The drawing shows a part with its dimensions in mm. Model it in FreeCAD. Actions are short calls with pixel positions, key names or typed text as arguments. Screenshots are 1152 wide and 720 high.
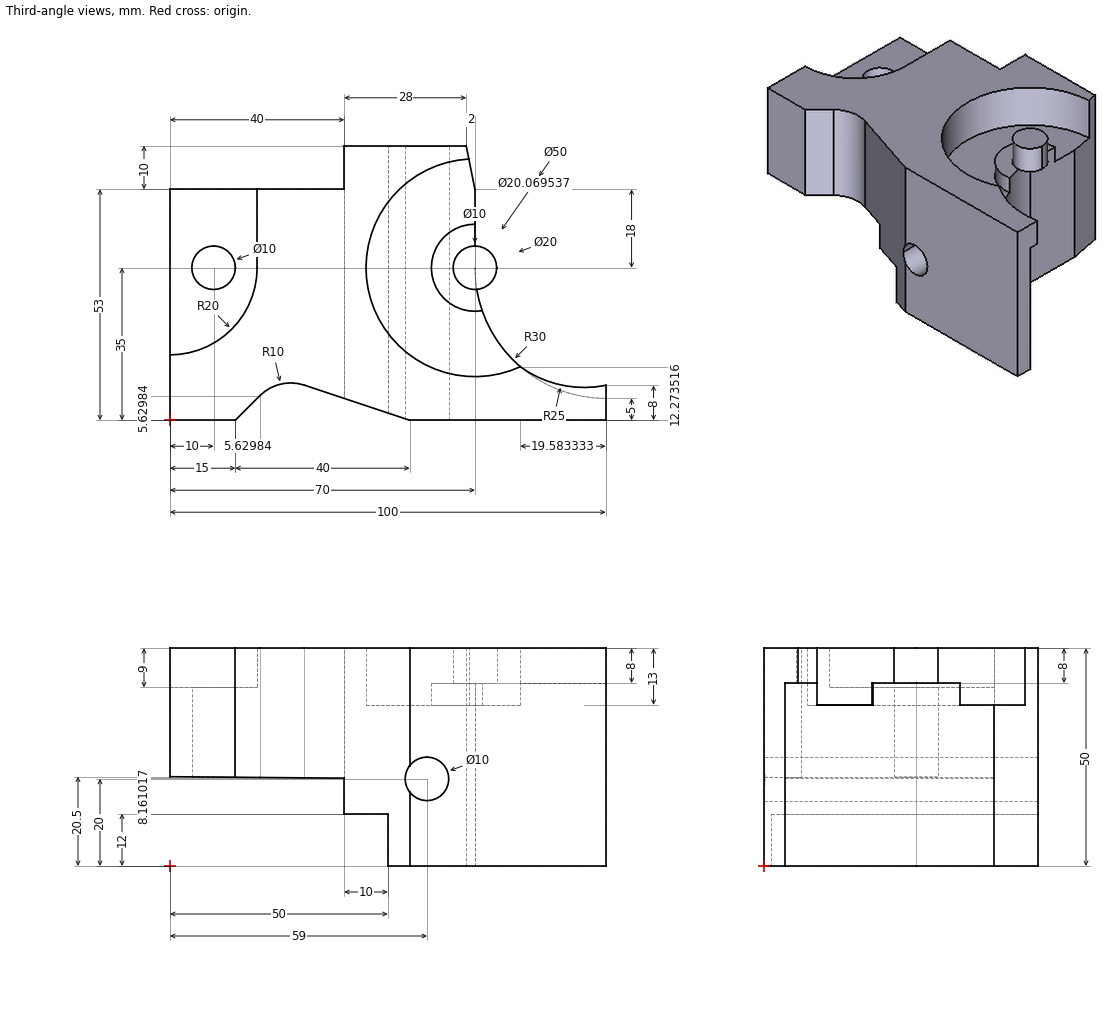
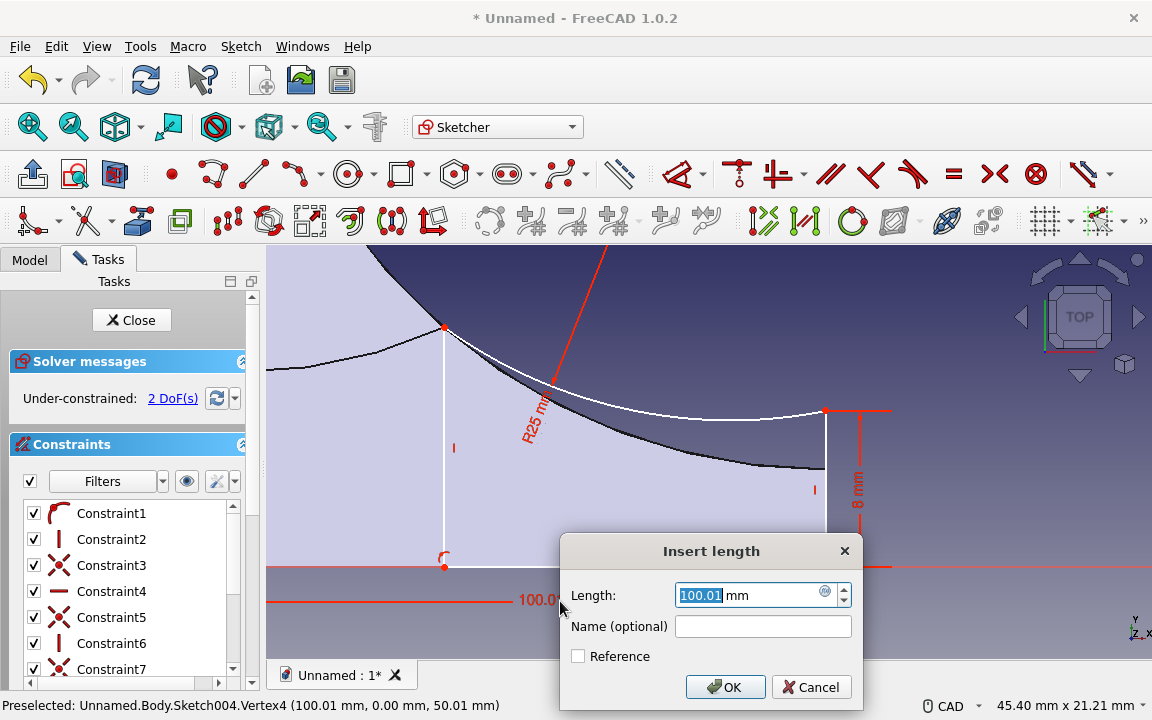
text(100)
key(Return)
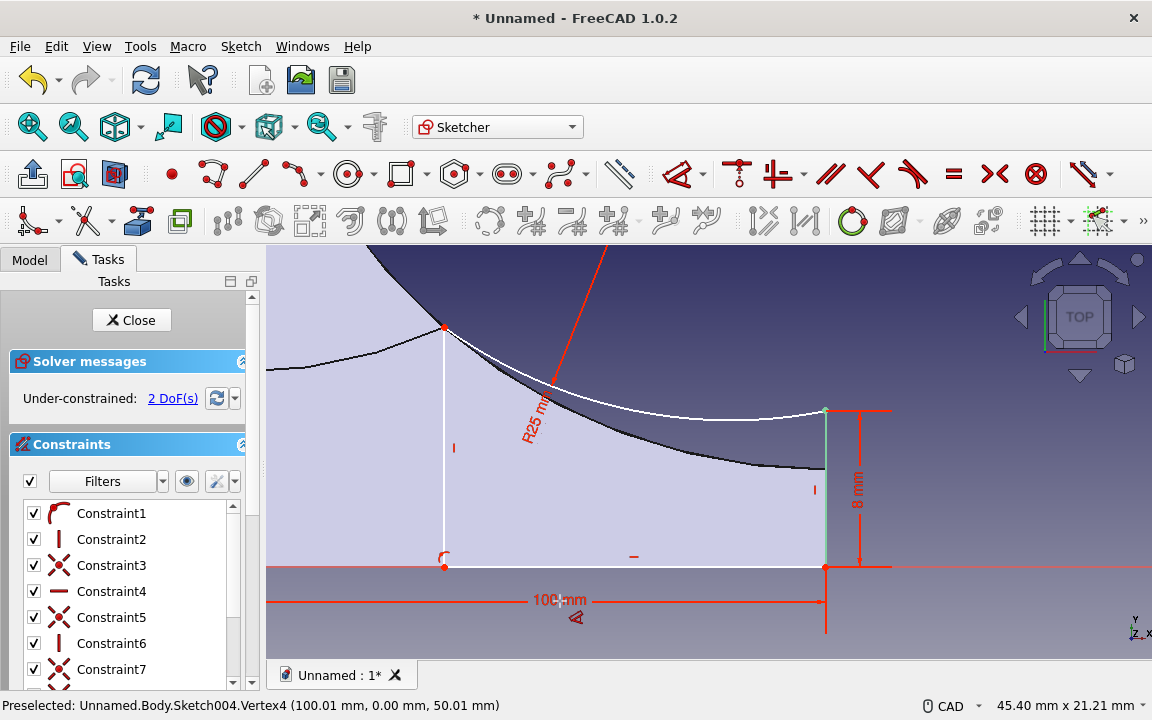
click(444, 399)
click(410, 447)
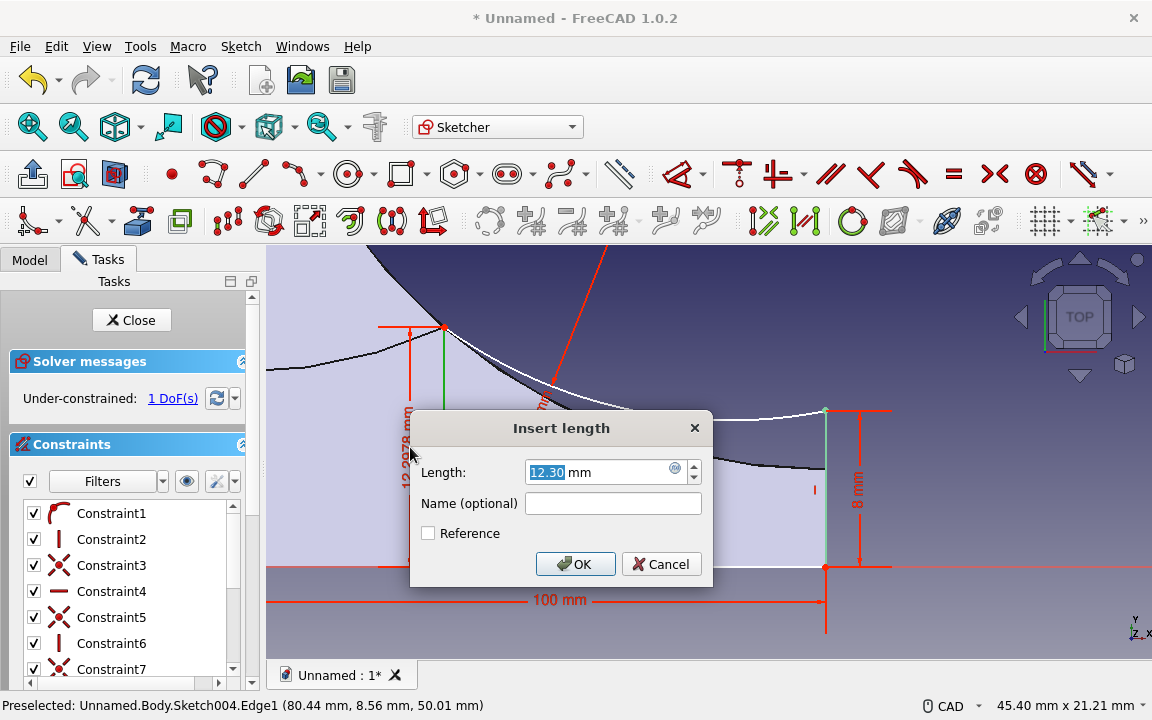
text(12.273516)
key(Return)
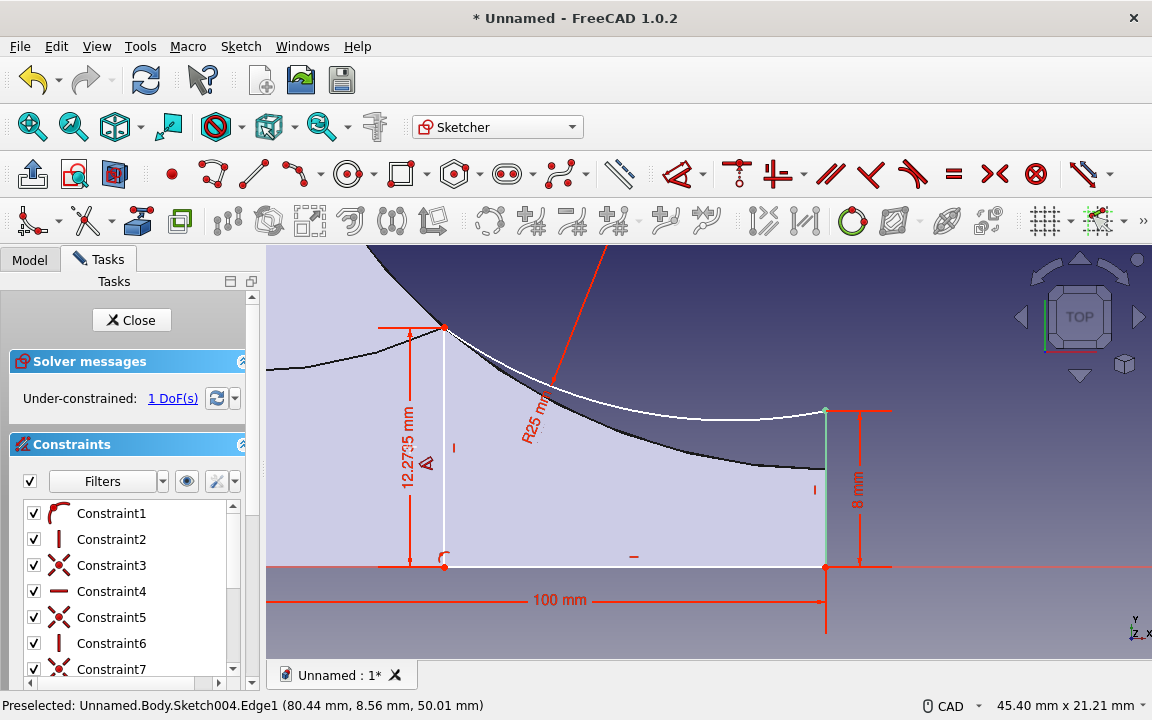
click(559, 567)
click(635, 601)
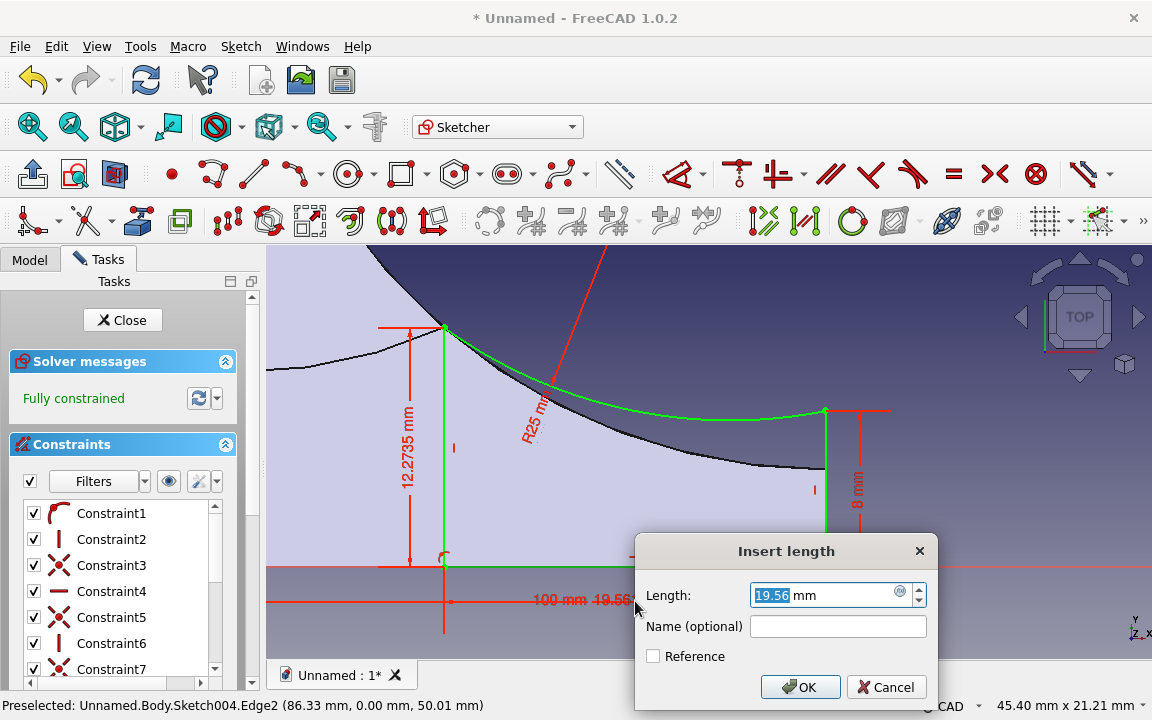
text(19.583333)
key(Return)
key(Escape)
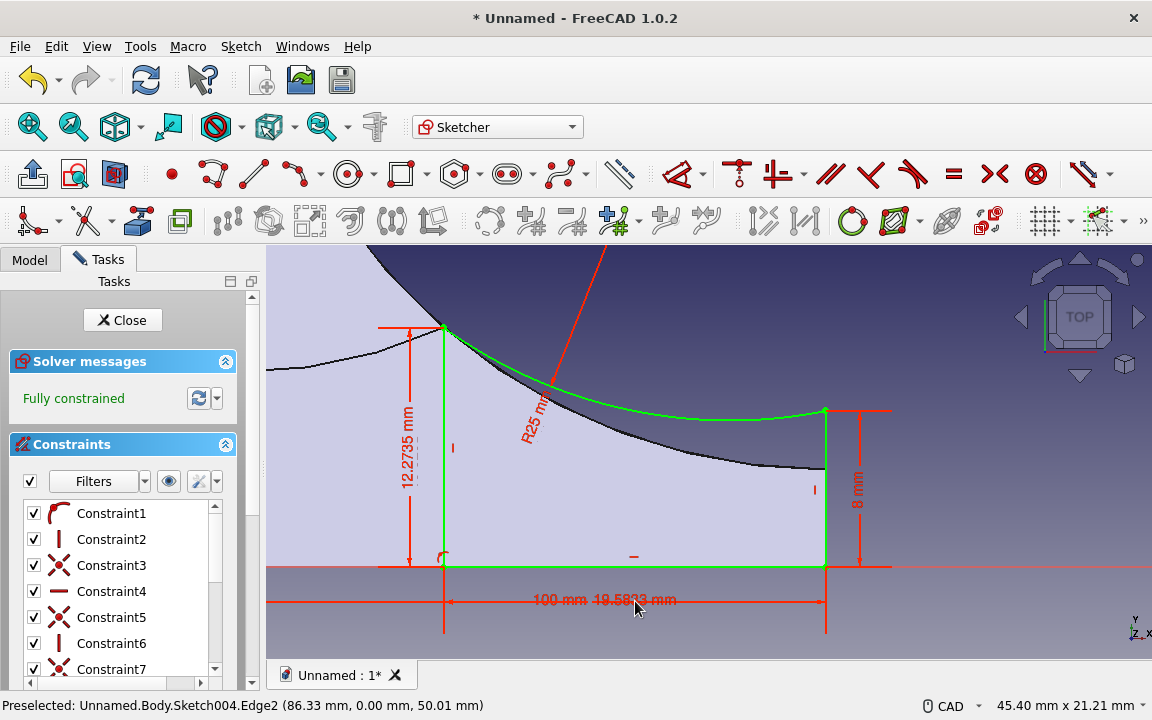
click(123, 320)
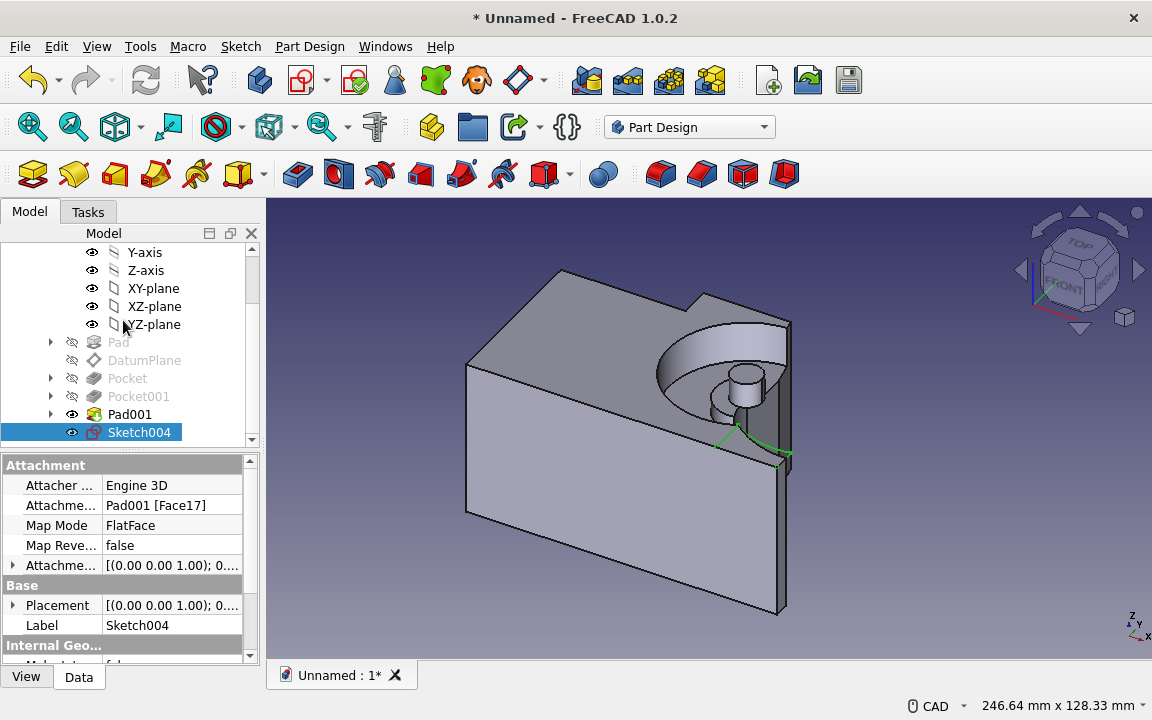
click(33, 174)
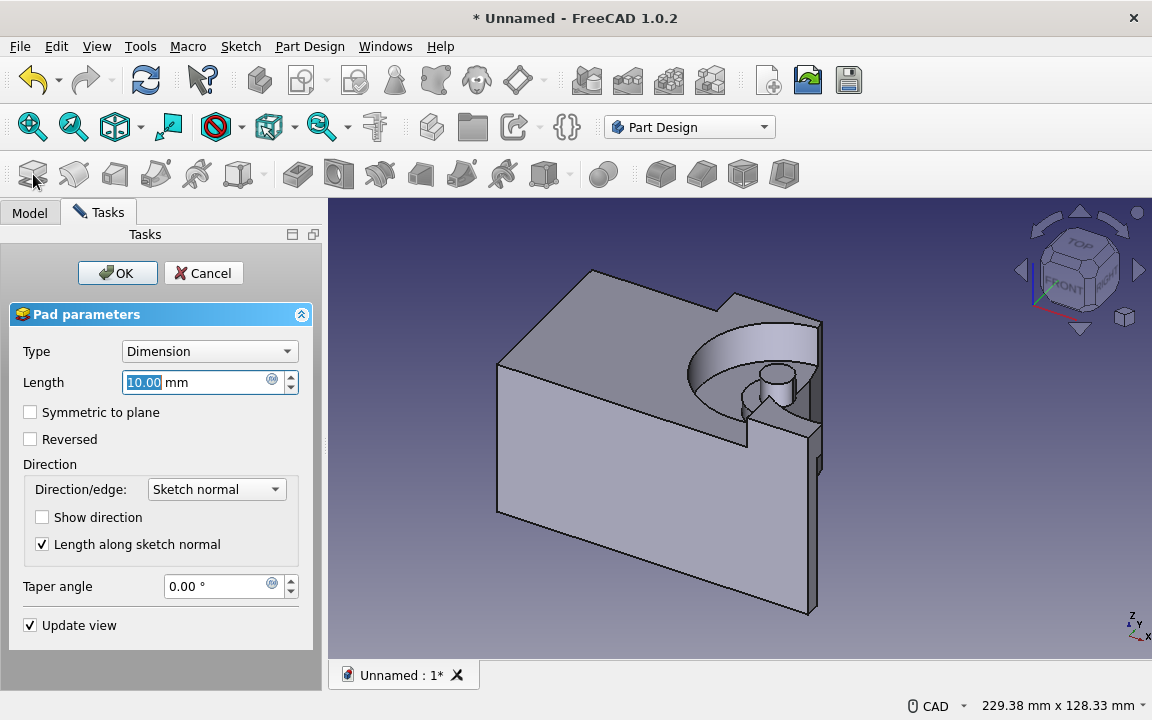
text(8)
key(Tab)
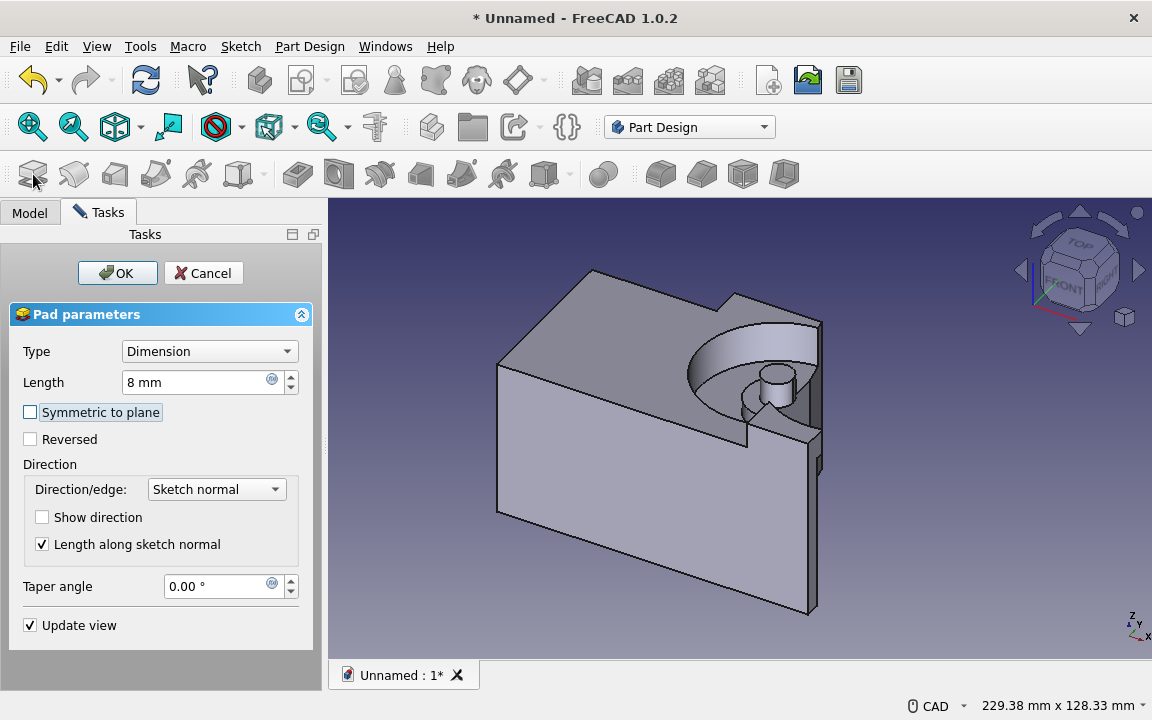
click(31, 439)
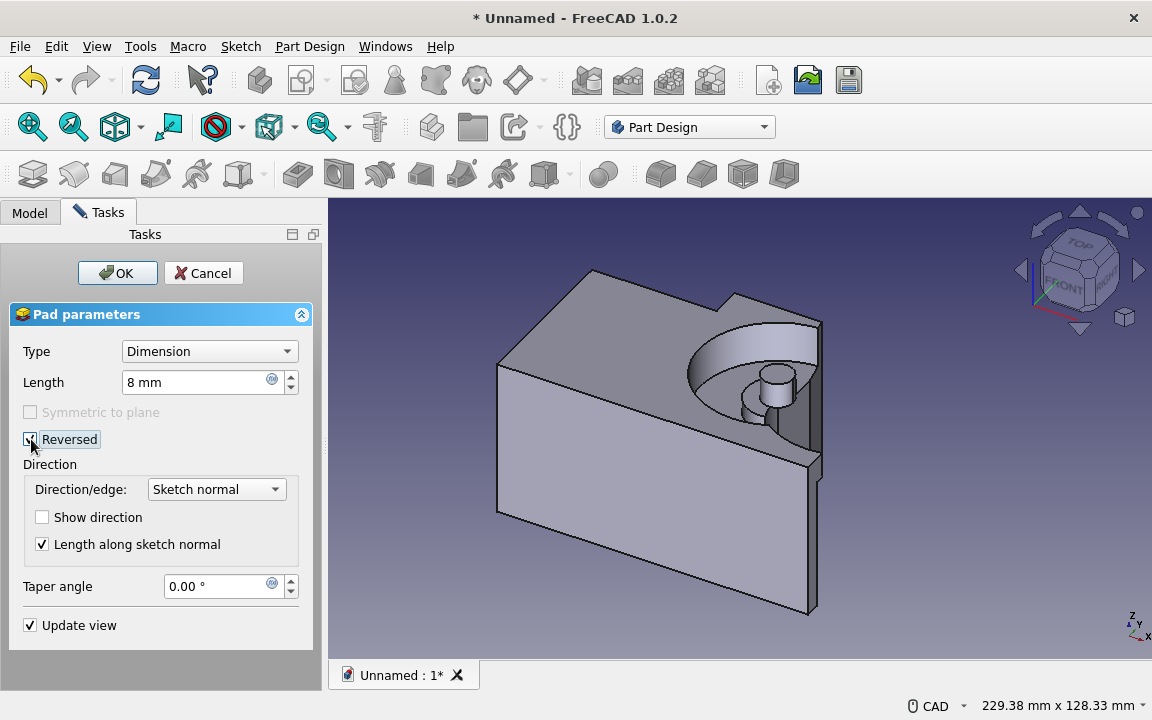
click(118, 273)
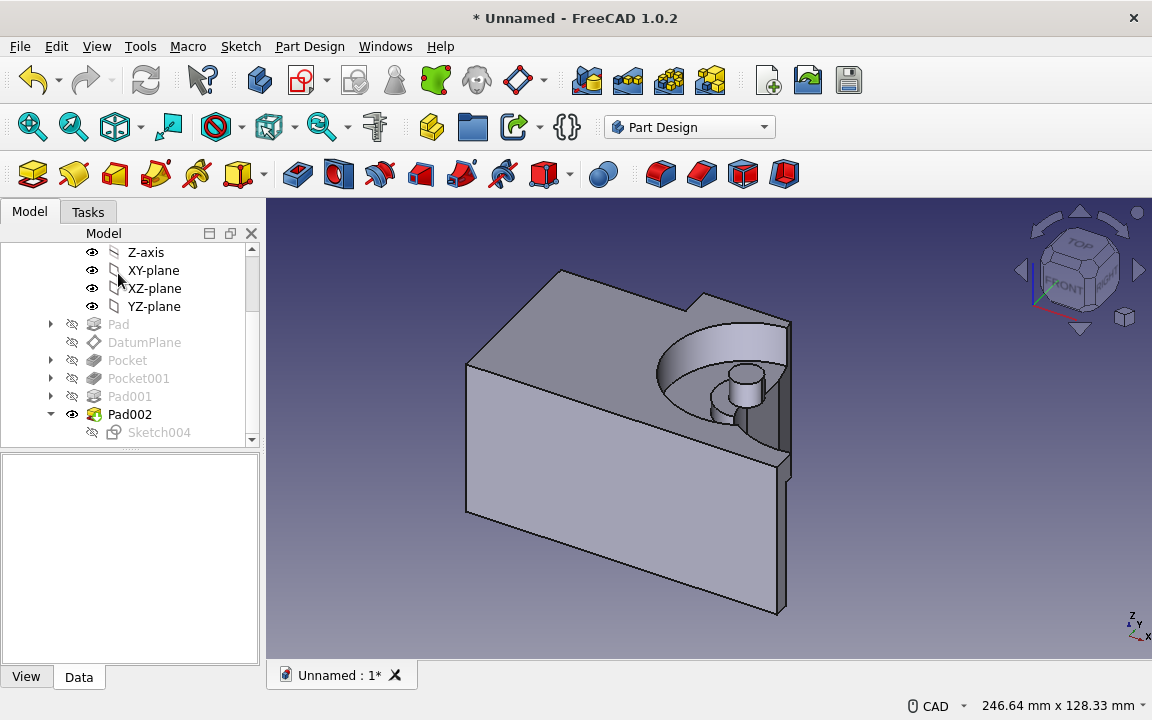
click(589, 329)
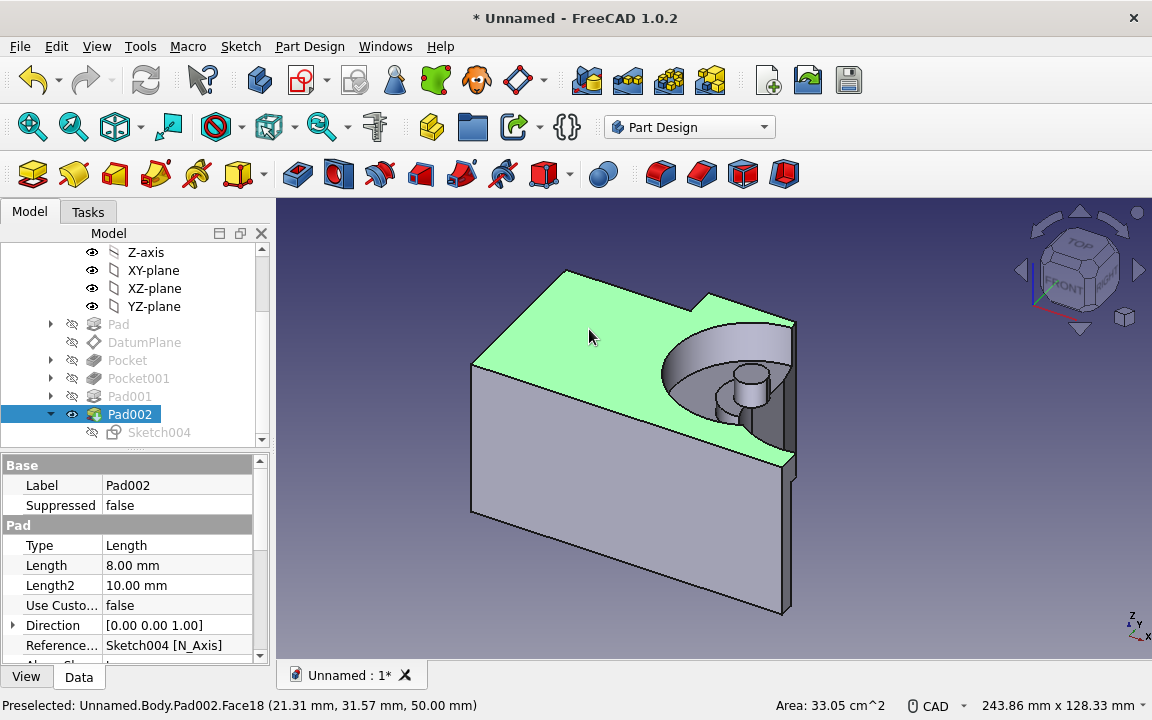
click(300, 80)